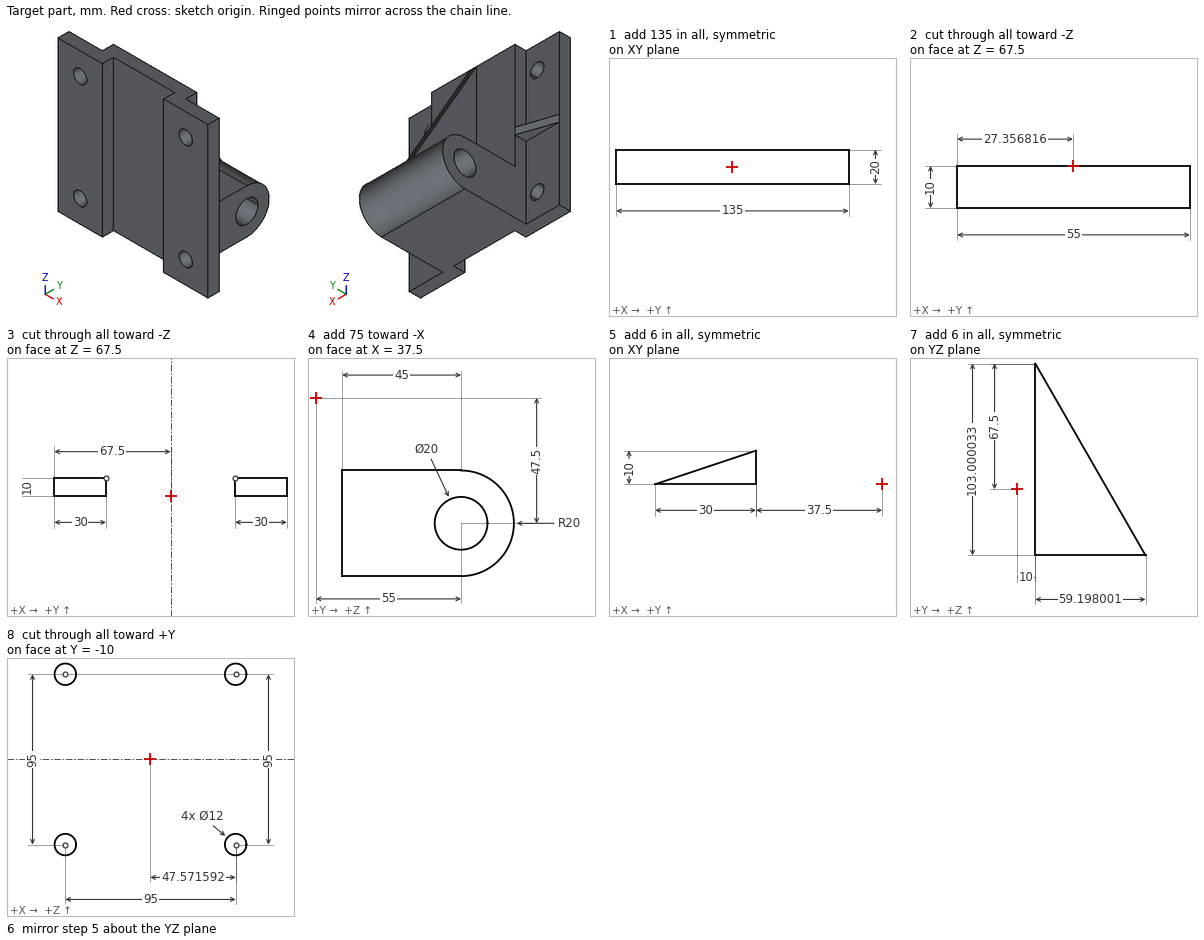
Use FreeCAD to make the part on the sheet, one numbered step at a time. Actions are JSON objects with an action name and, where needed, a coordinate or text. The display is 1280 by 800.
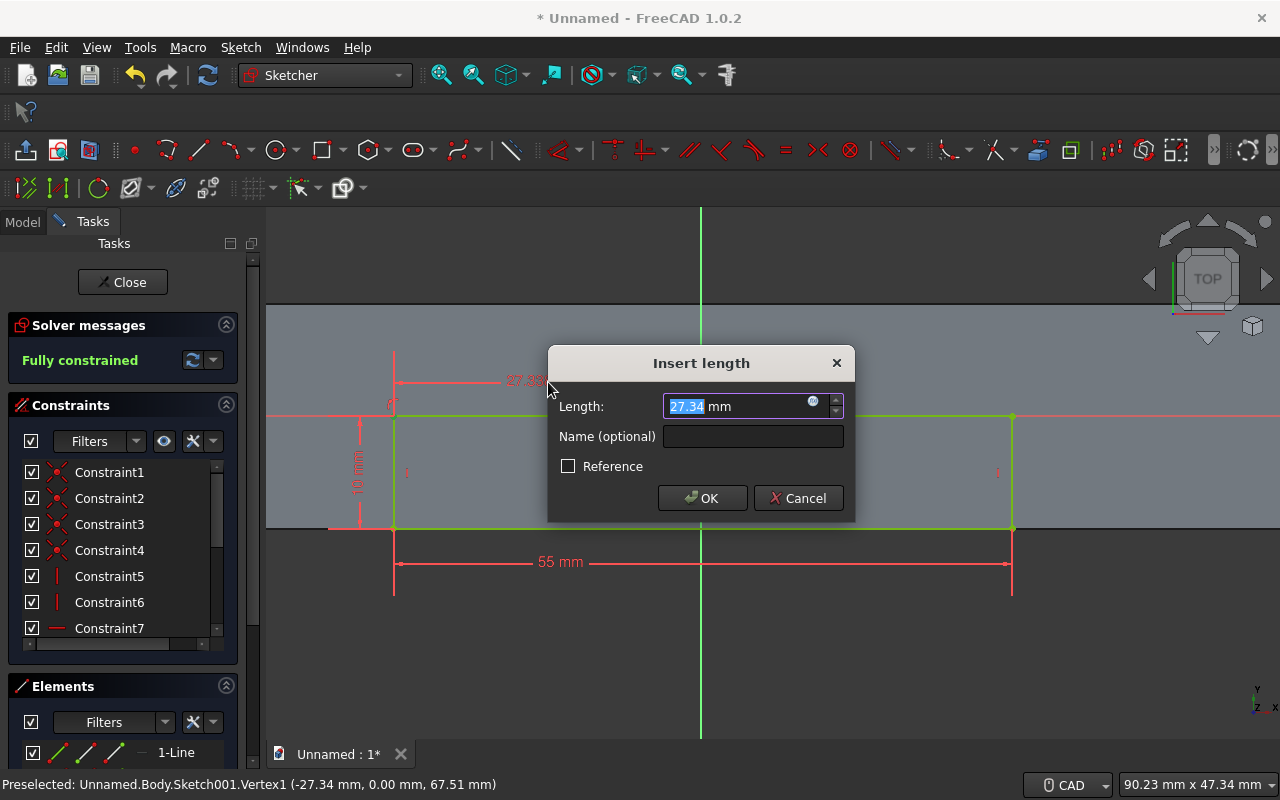
{"action": "type", "text": "27.356816"}
{"action": "key", "text": "Return"}
{"action": "key", "text": "Escape"}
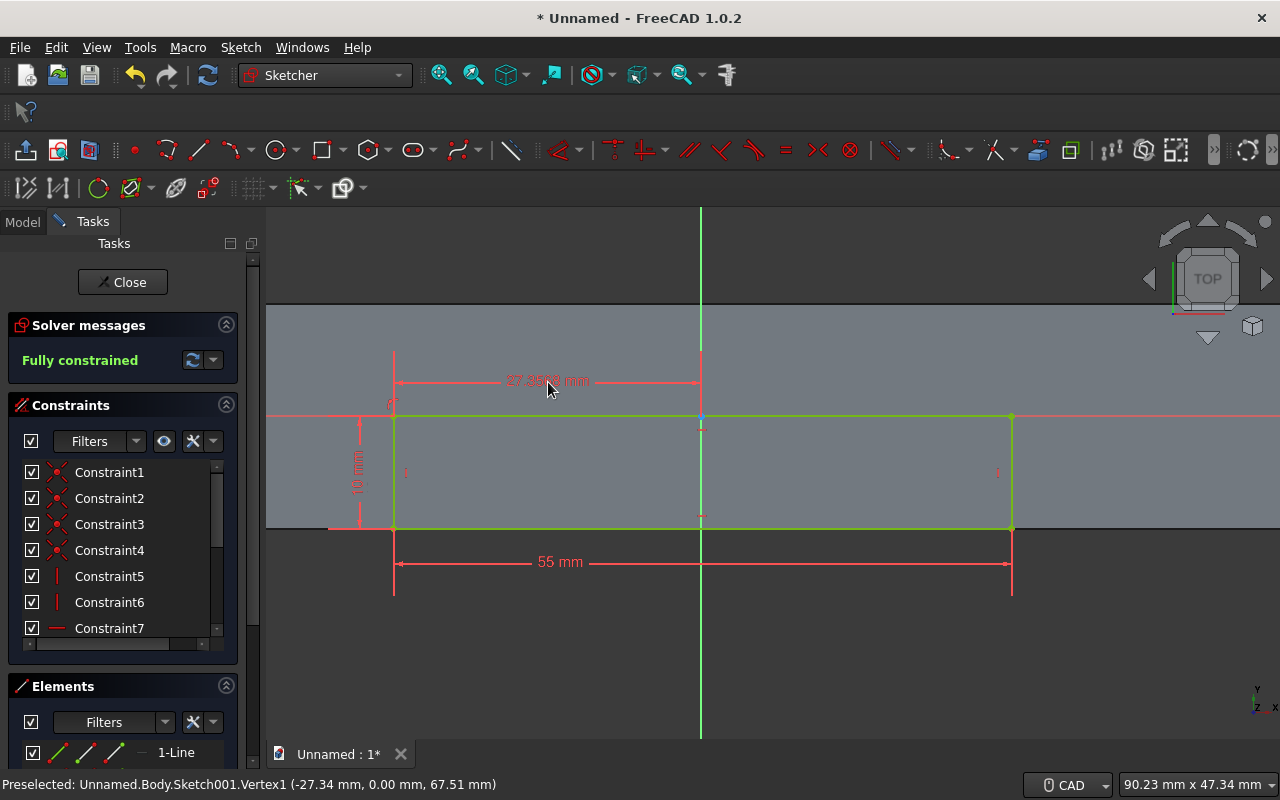
{"action": "left_click", "coordinate": [123, 282]}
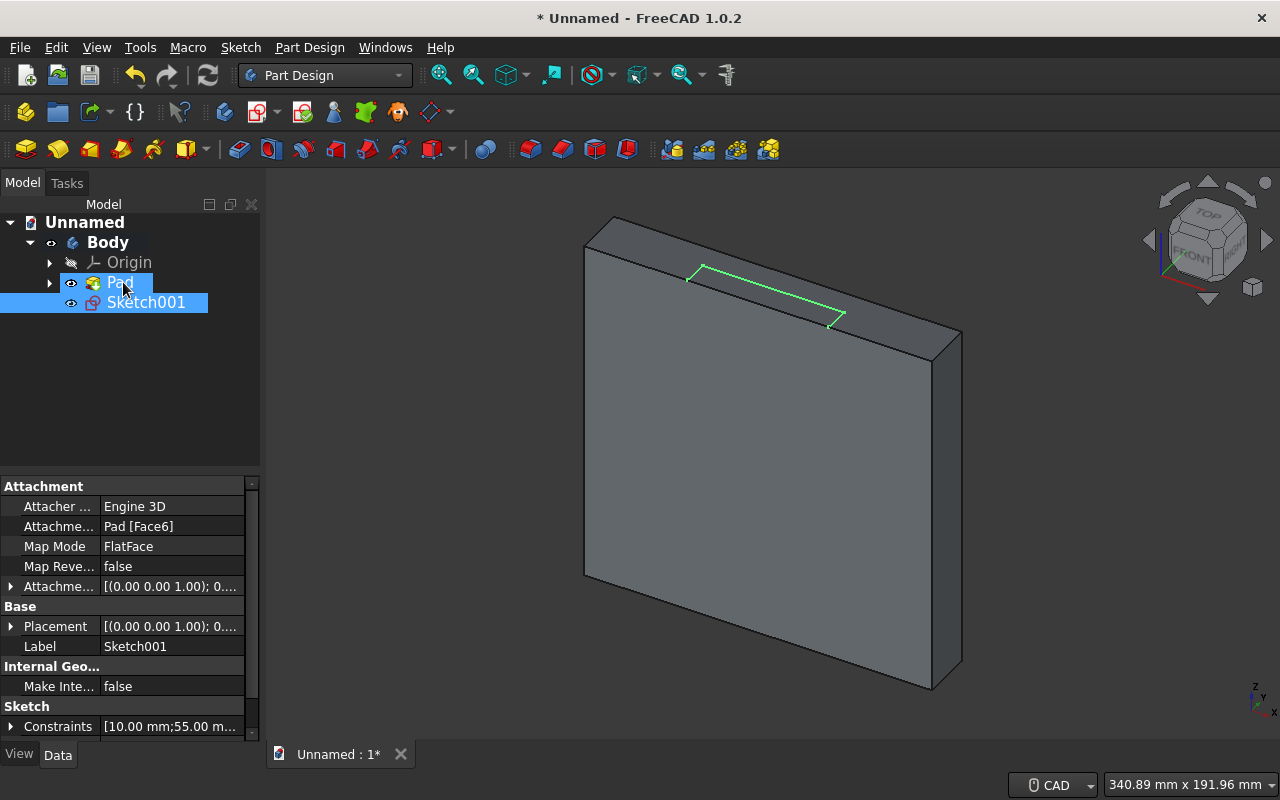
{"action": "left_click", "coordinate": [240, 150]}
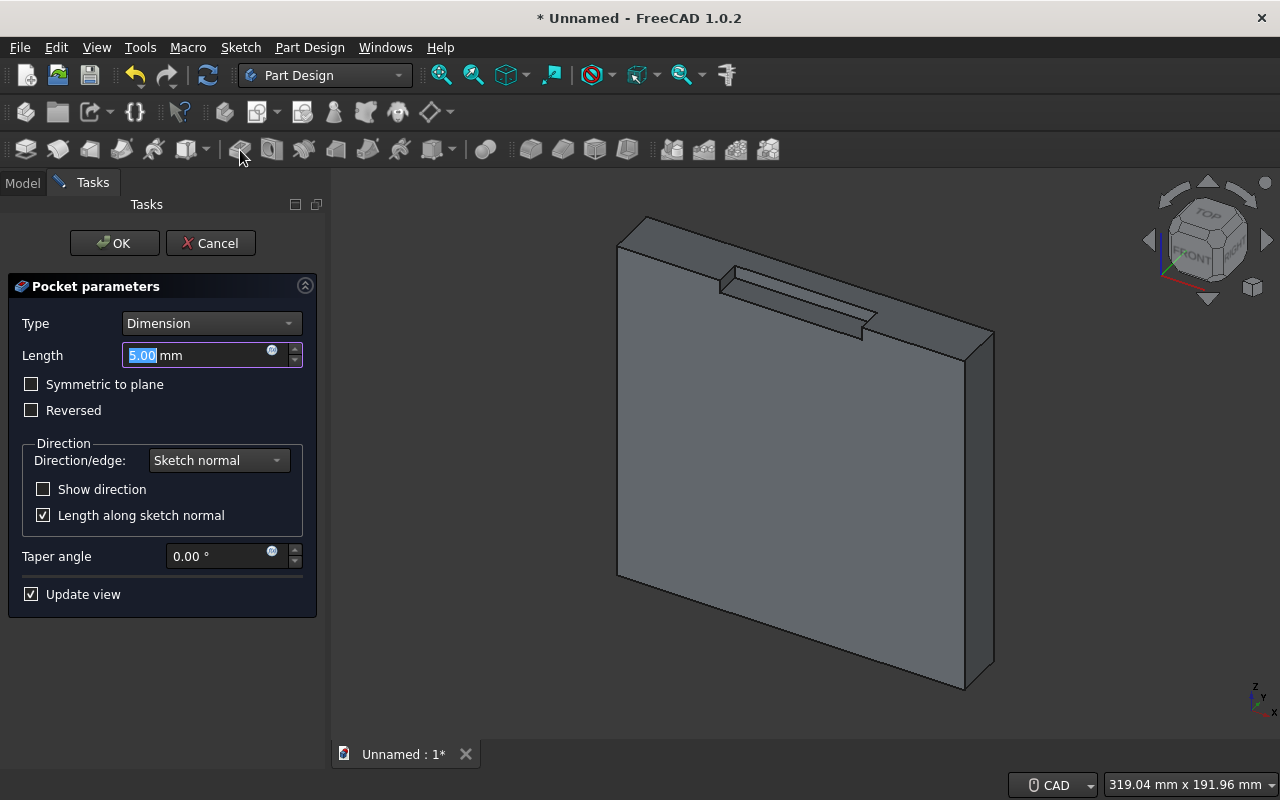
{"action": "left_click", "coordinate": [212, 324]}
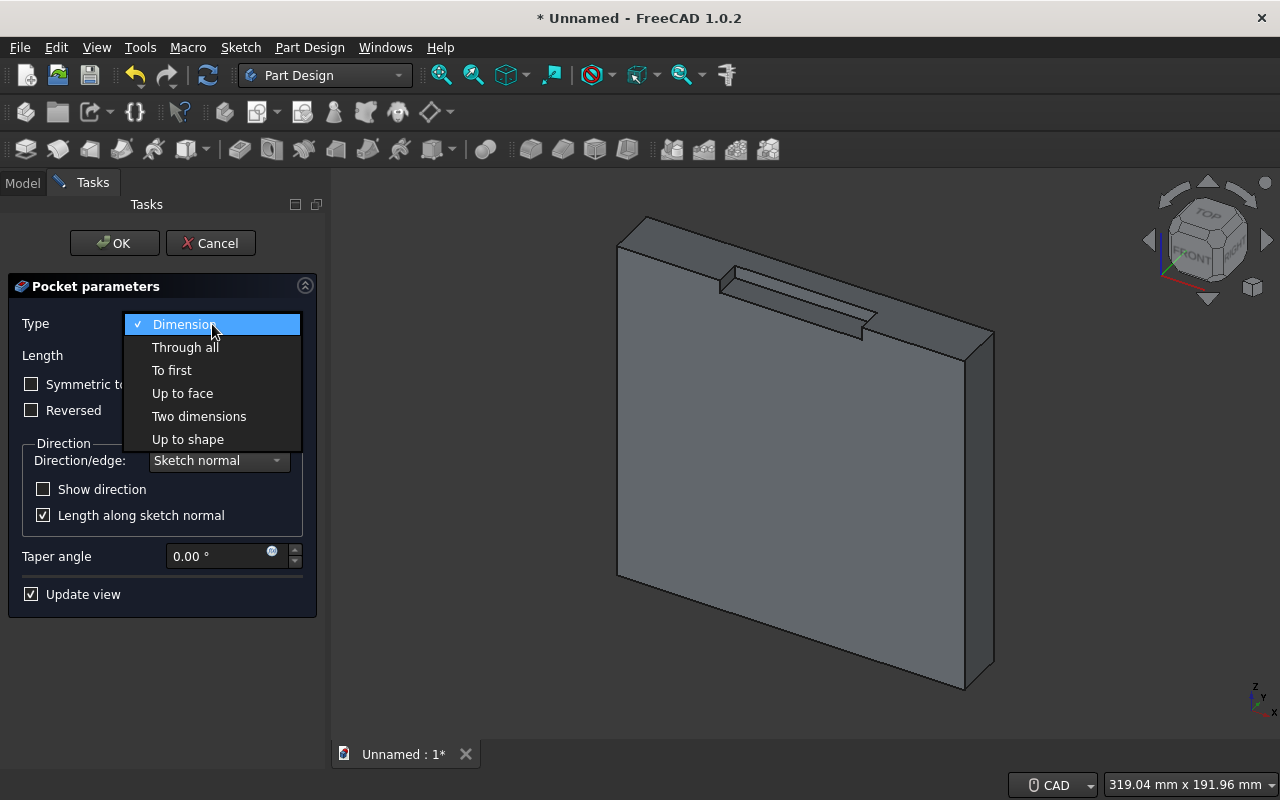
{"action": "left_click", "coordinate": [212, 348]}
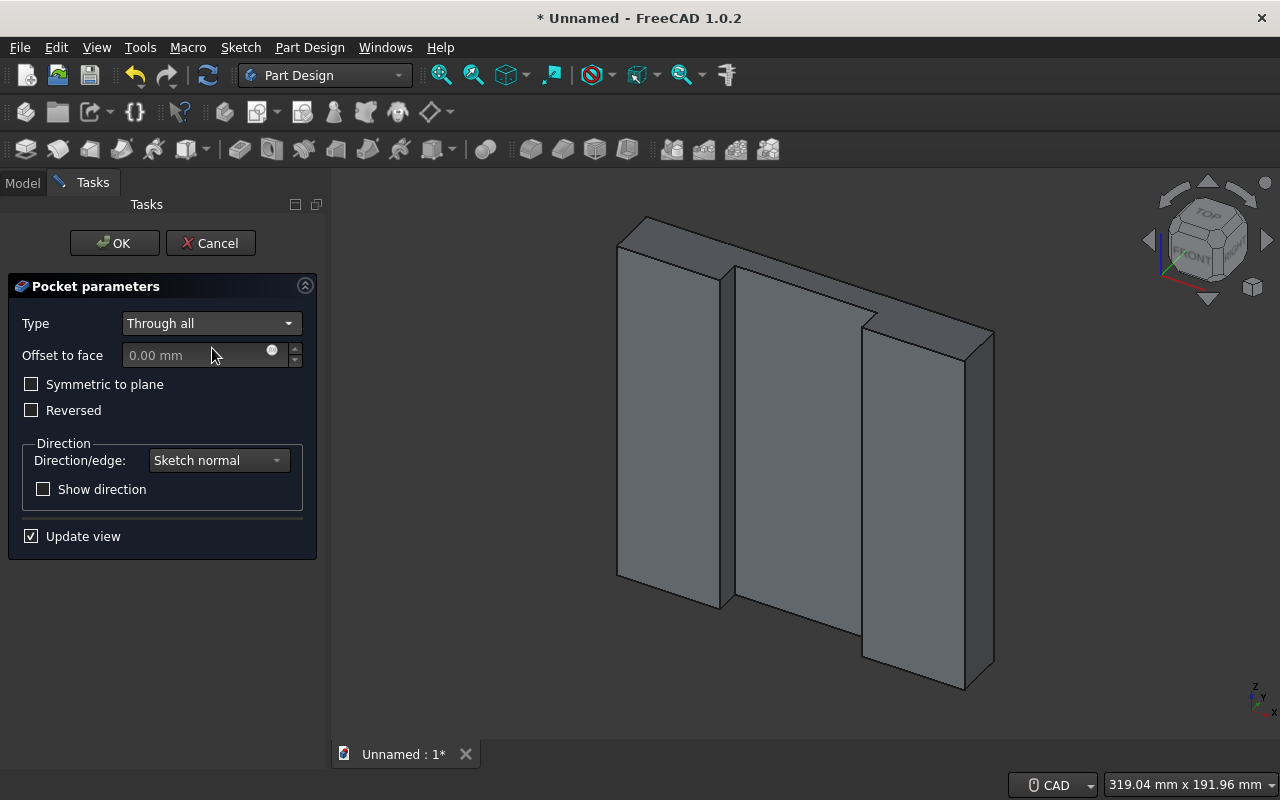
{"action": "left_click", "coordinate": [115, 243]}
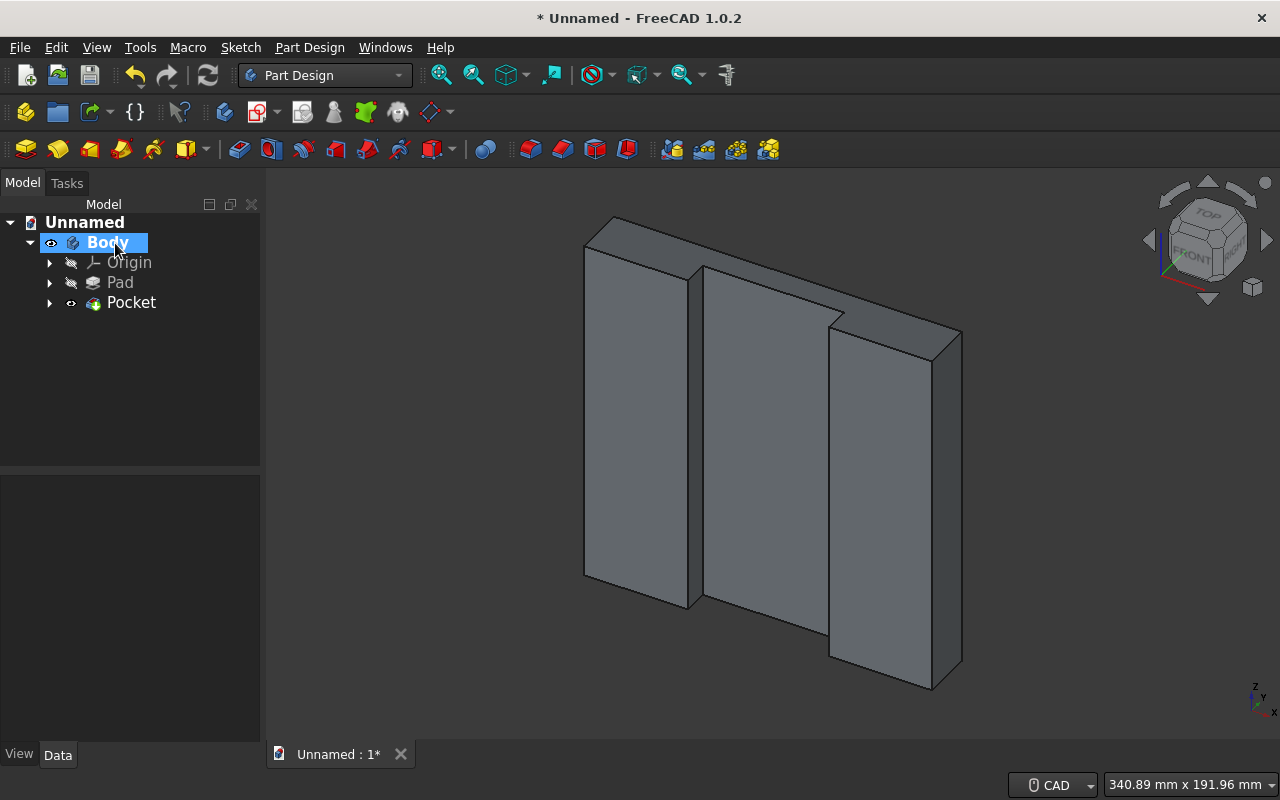
{"action": "left_click", "coordinate": [872, 321]}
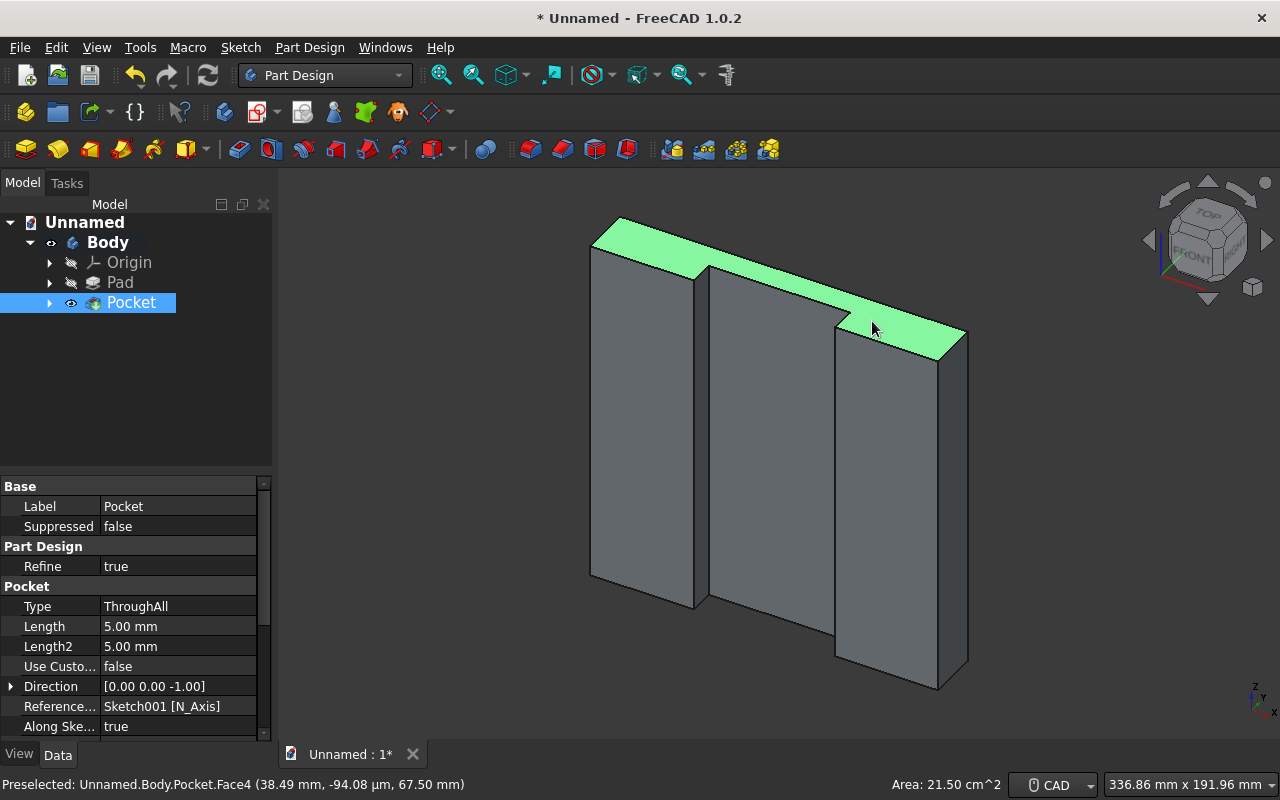
{"action": "left_click", "coordinate": [258, 112]}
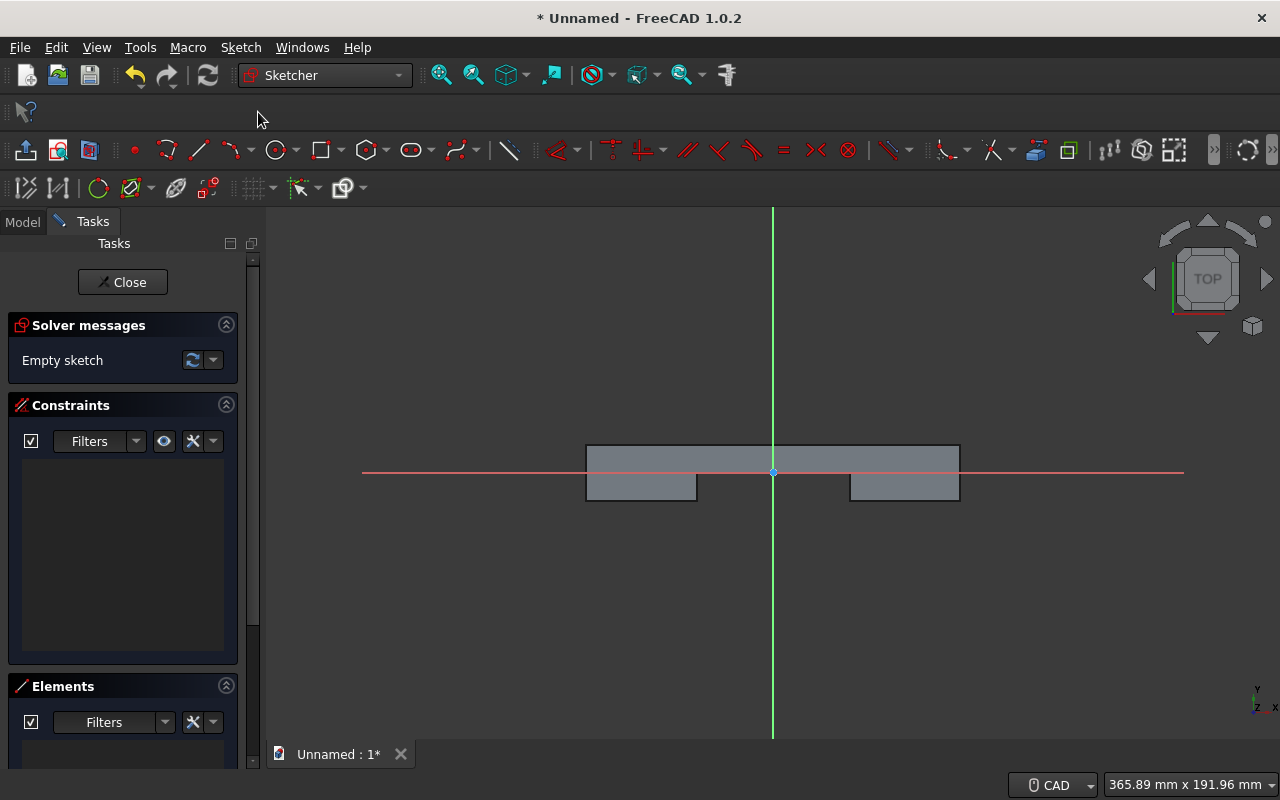
{"action": "scroll", "coordinate": [912, 431], "scroll_direction": "up", "scroll_amount": 2}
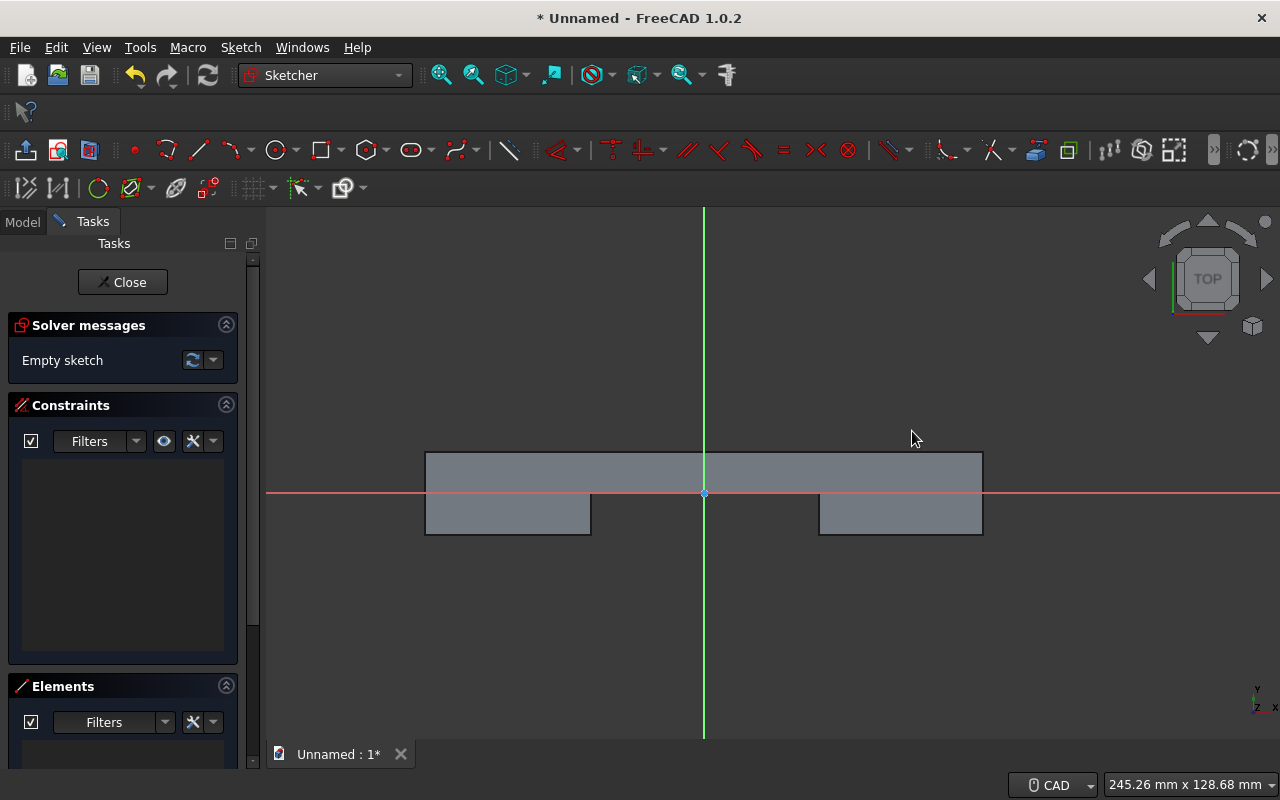
{"action": "left_click", "coordinate": [322, 150]}